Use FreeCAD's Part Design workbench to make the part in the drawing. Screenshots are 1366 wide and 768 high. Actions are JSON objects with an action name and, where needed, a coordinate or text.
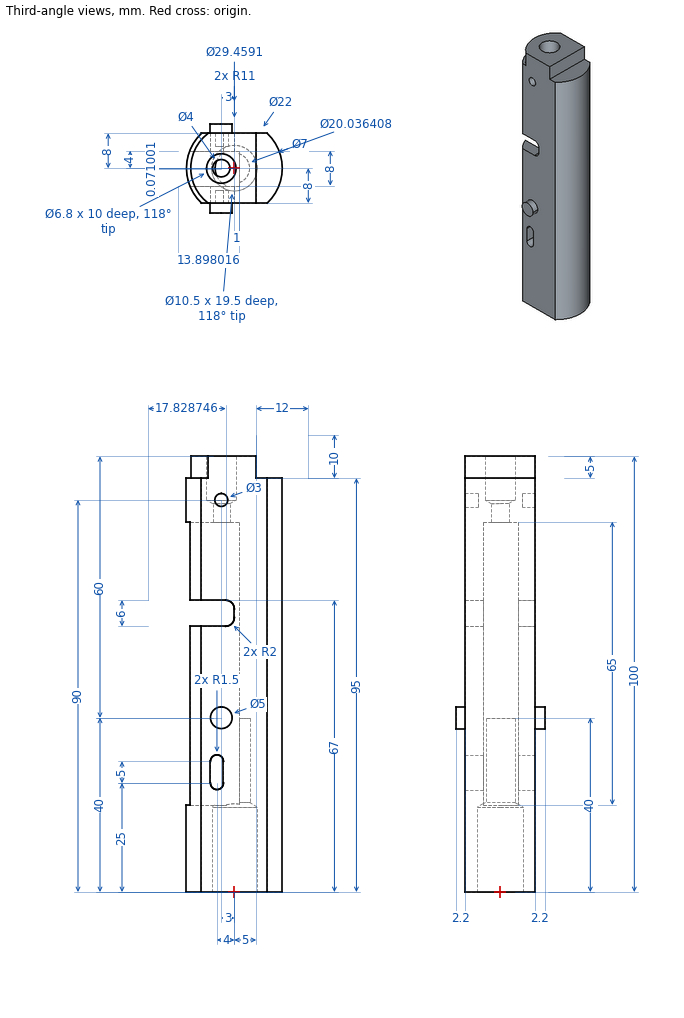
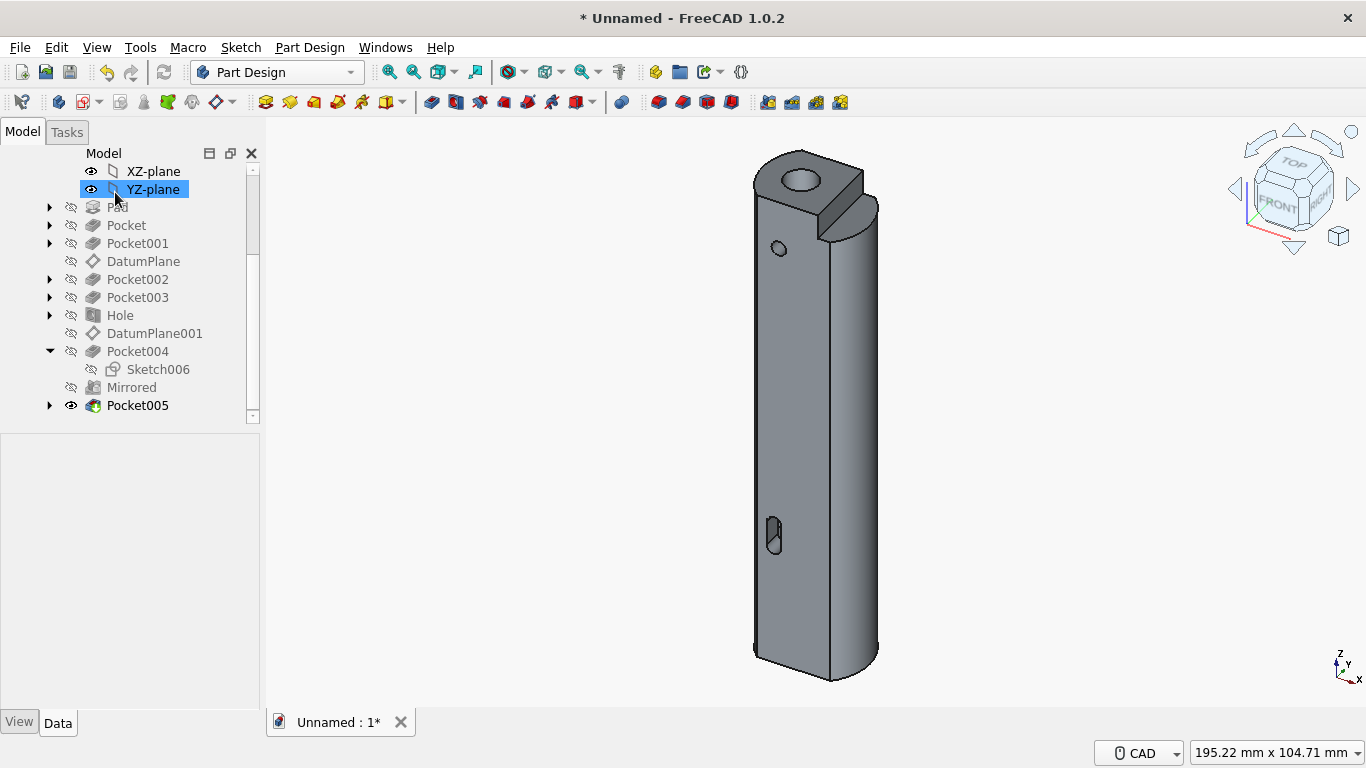
{"action": "scroll", "coordinate": [160, 293], "scroll_direction": "down", "scroll_amount": 3}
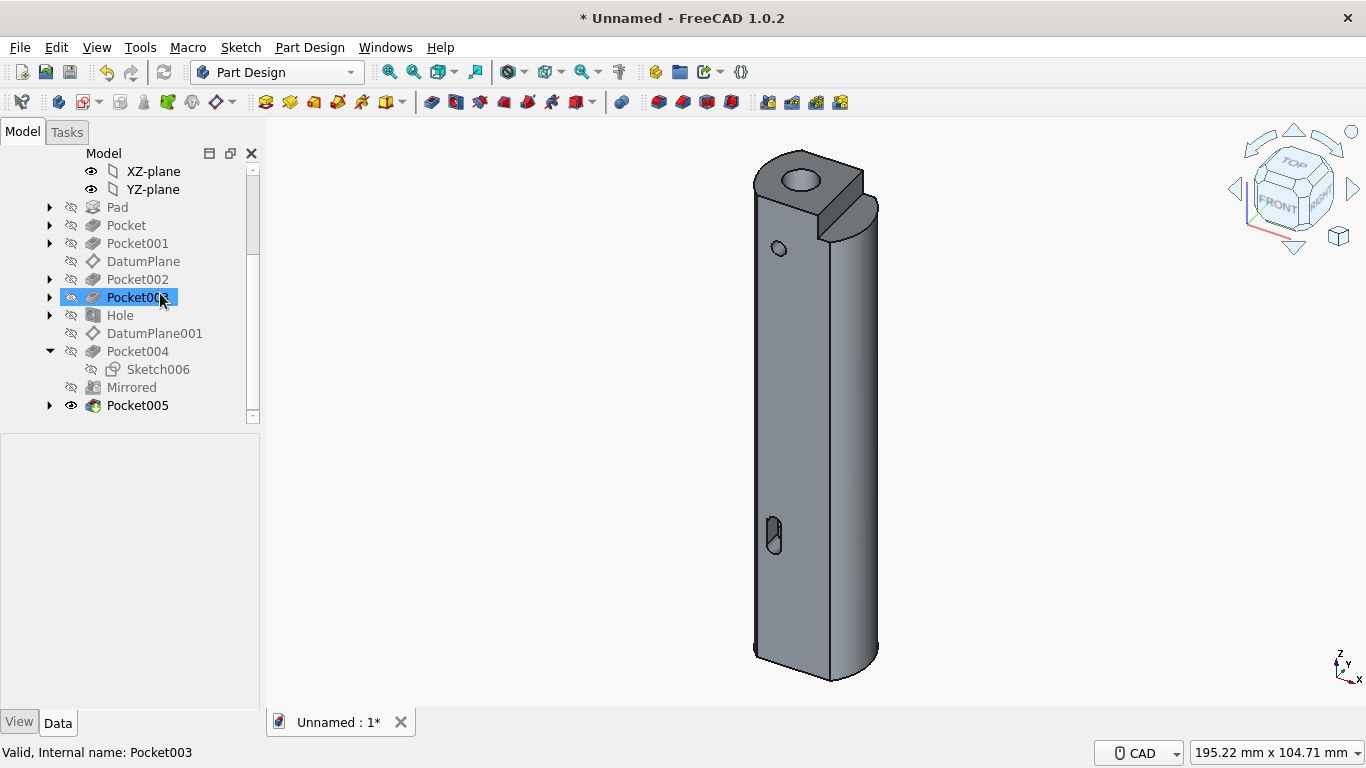
{"action": "scroll", "coordinate": [160, 293], "scroll_direction": "up", "scroll_amount": 15}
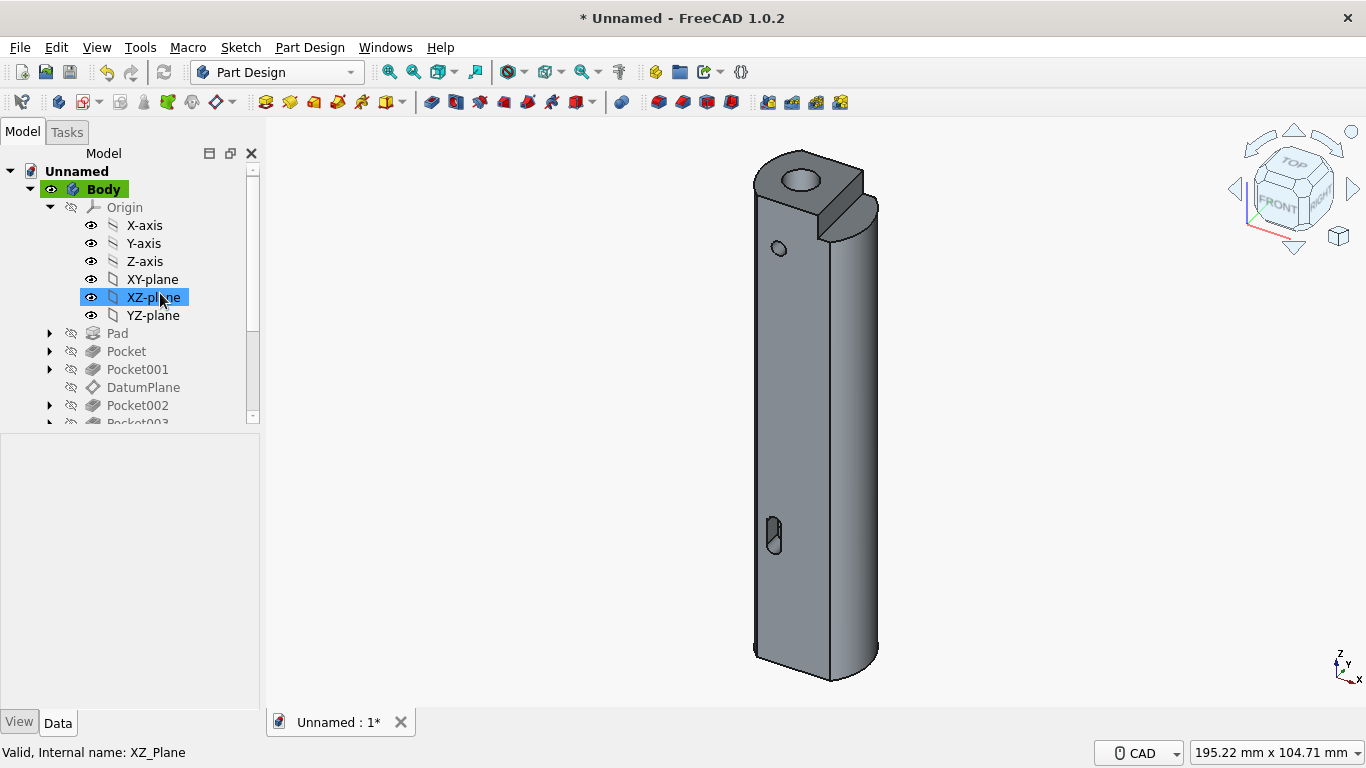
{"action": "left_click", "coordinate": [136, 297]}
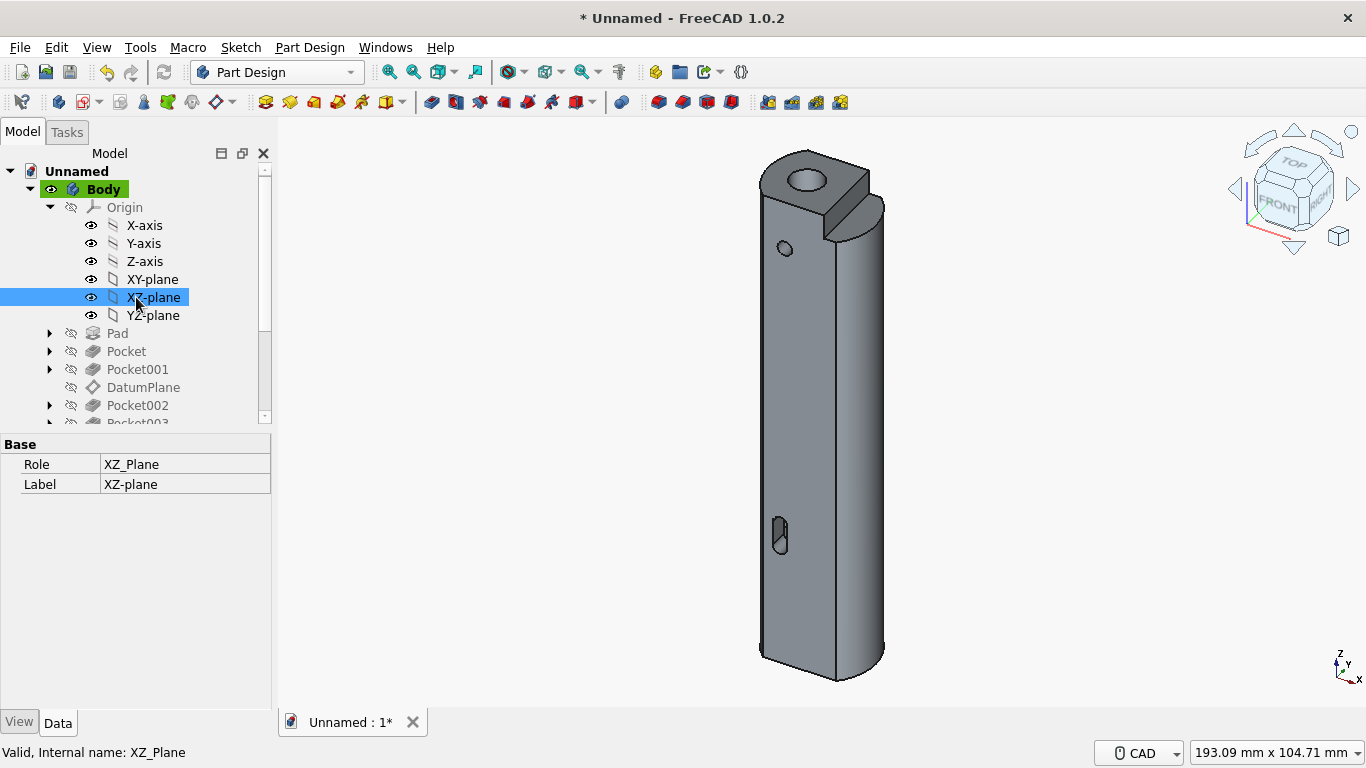
{"action": "left_click", "coordinate": [216, 102]}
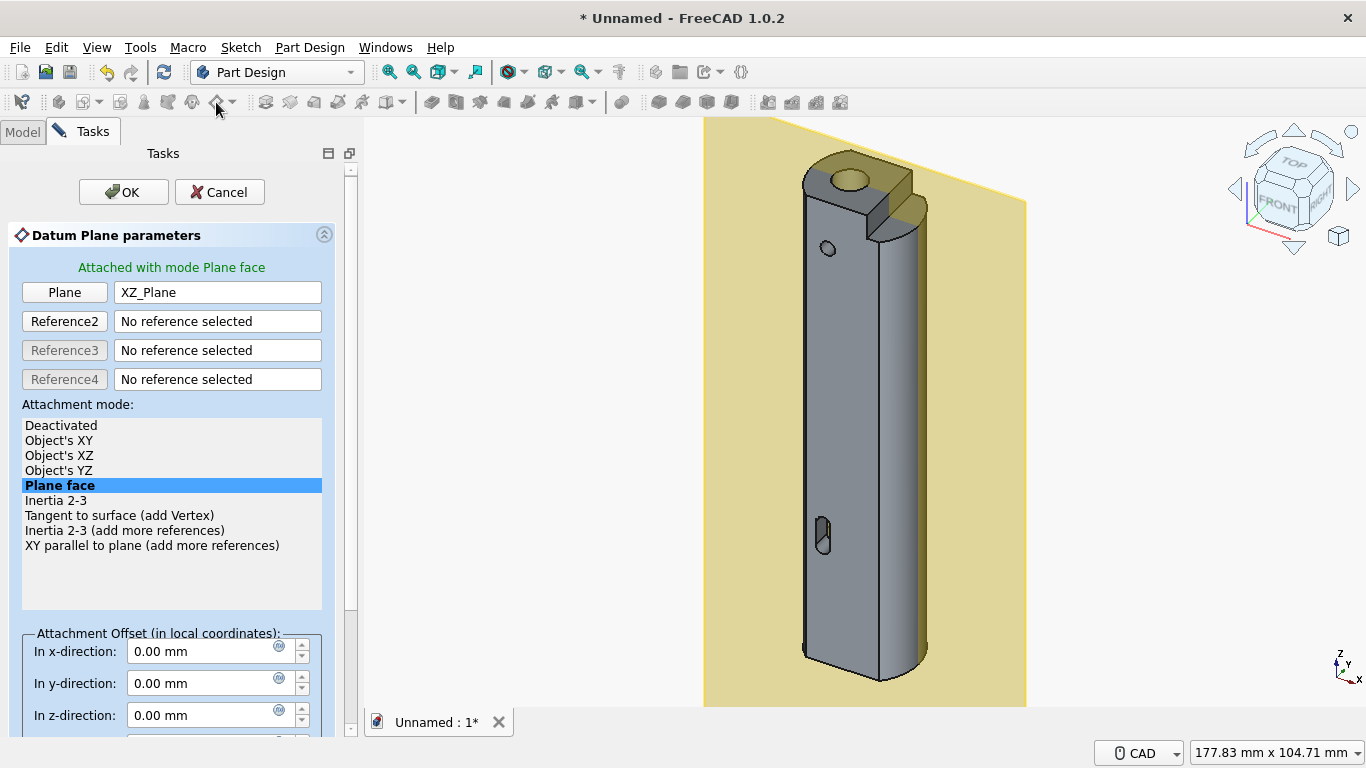
{"action": "triple_click", "coordinate": [210, 715]}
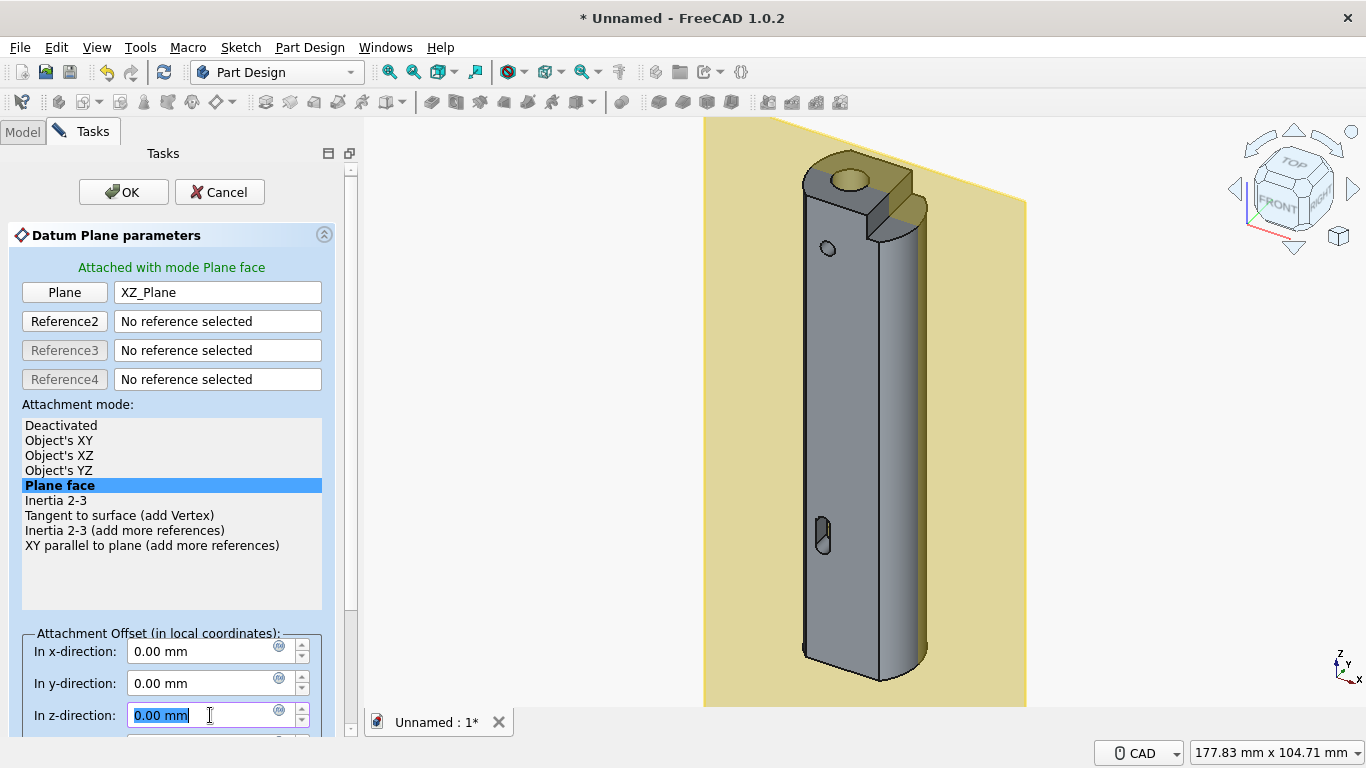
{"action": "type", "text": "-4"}
{"action": "key", "text": "Tab"}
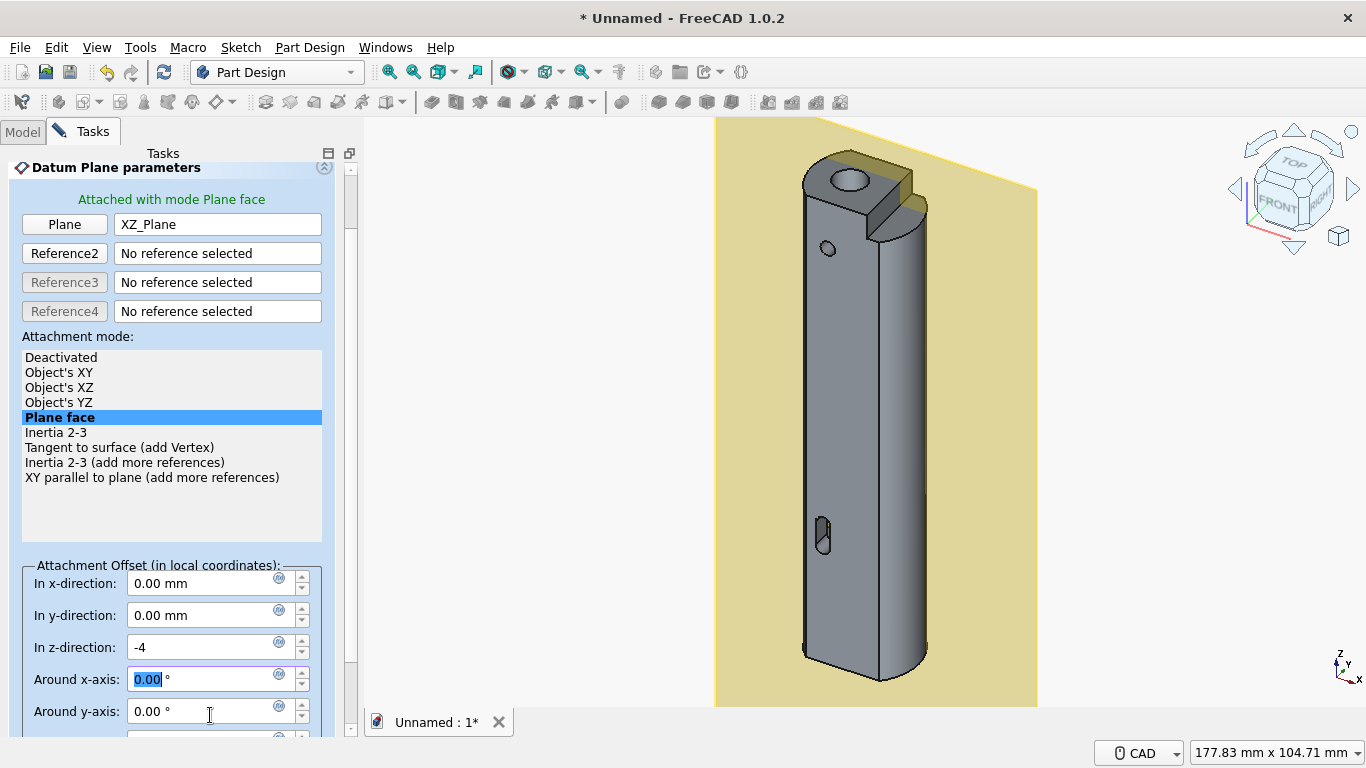
{"action": "scroll", "coordinate": [351, 450], "scroll_direction": "up", "scroll_amount": 2}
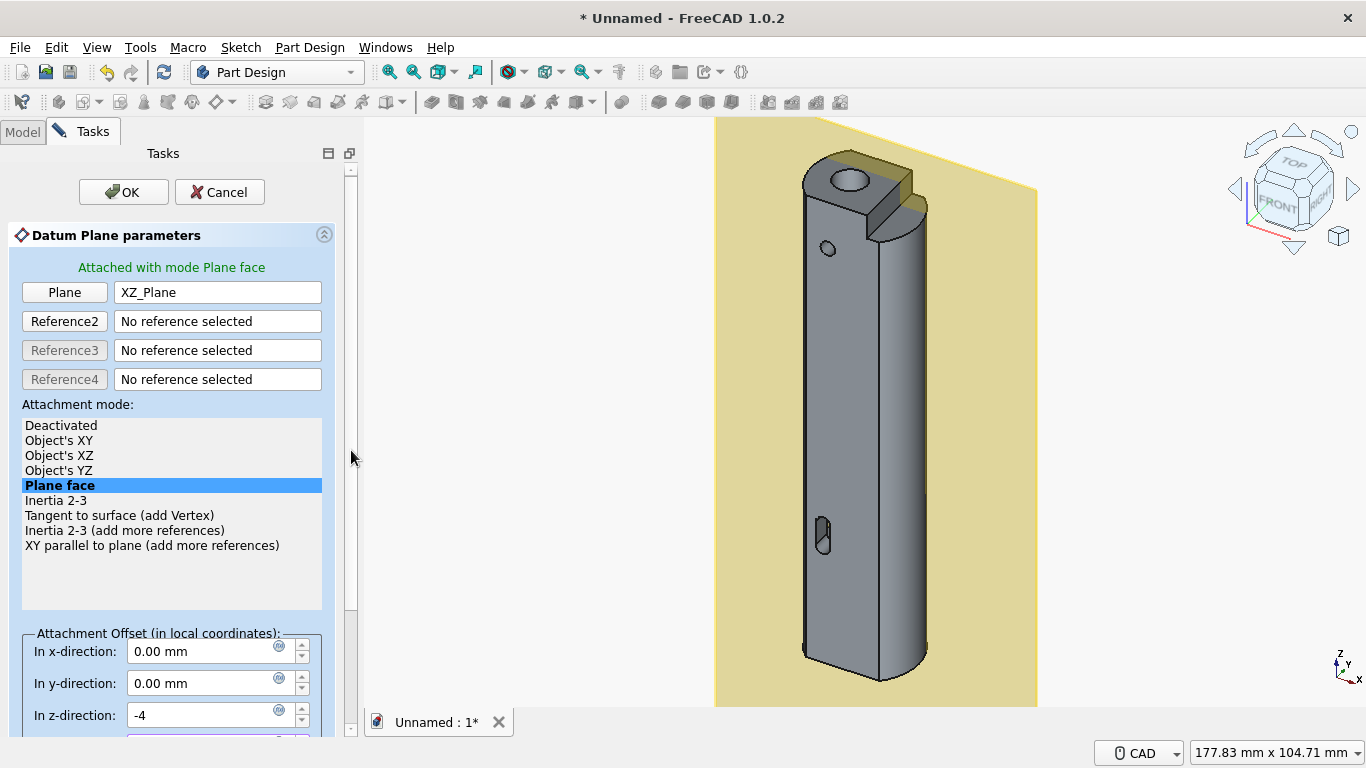
{"action": "left_click", "coordinate": [124, 192]}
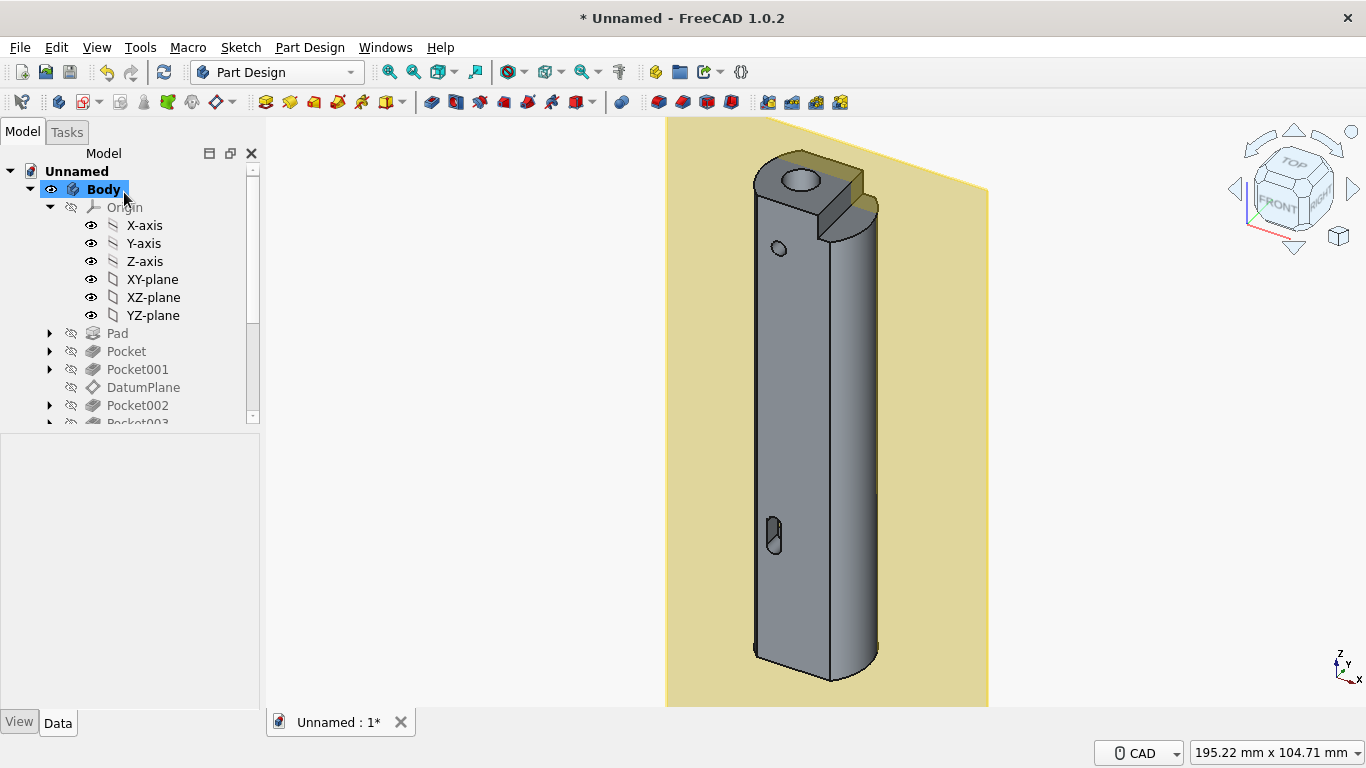
{"action": "scroll", "coordinate": [100, 293], "scroll_direction": "down", "scroll_amount": 3}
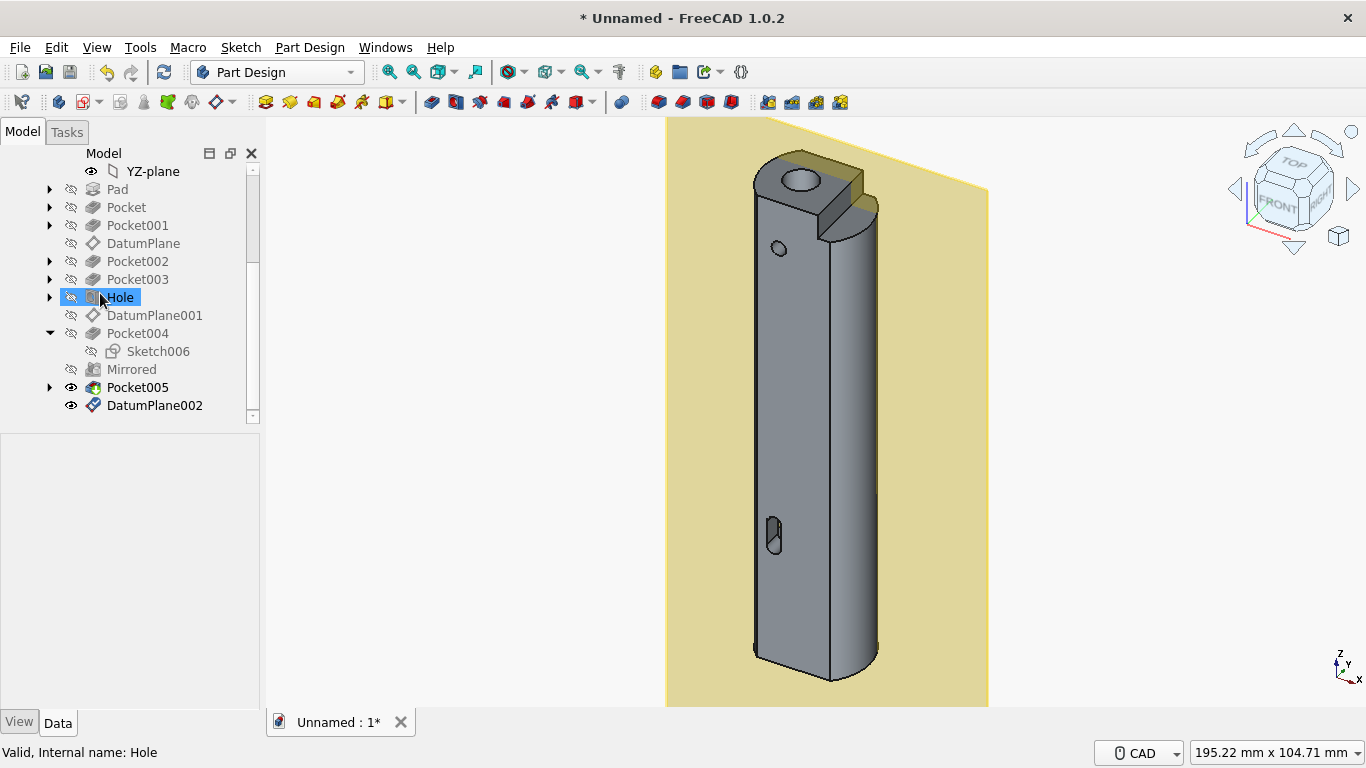
{"action": "left_click", "coordinate": [116, 405]}